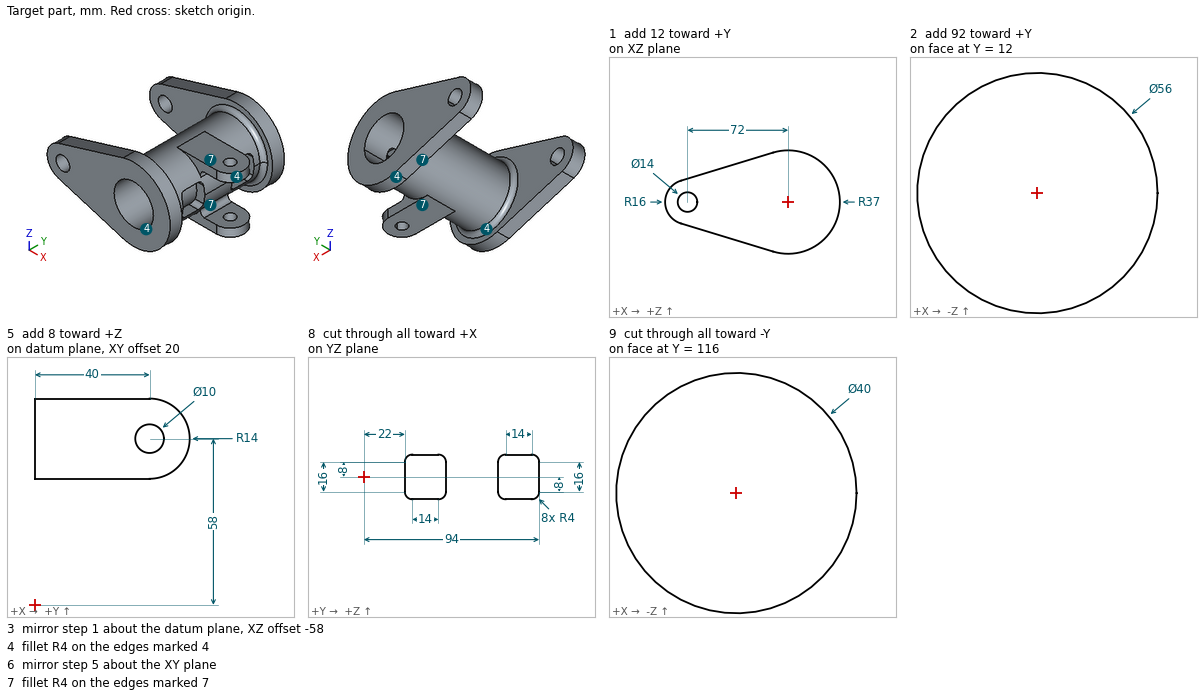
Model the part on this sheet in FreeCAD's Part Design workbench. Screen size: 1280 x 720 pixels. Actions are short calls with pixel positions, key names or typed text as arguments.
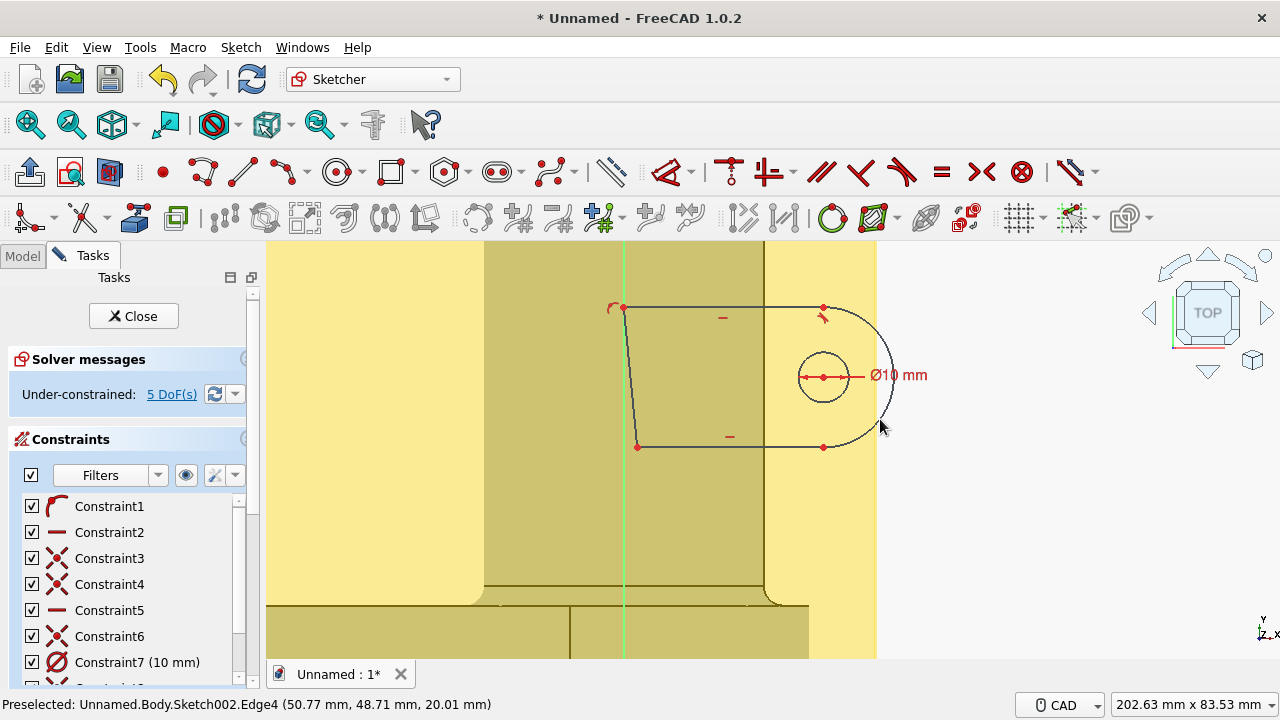
click(693, 447)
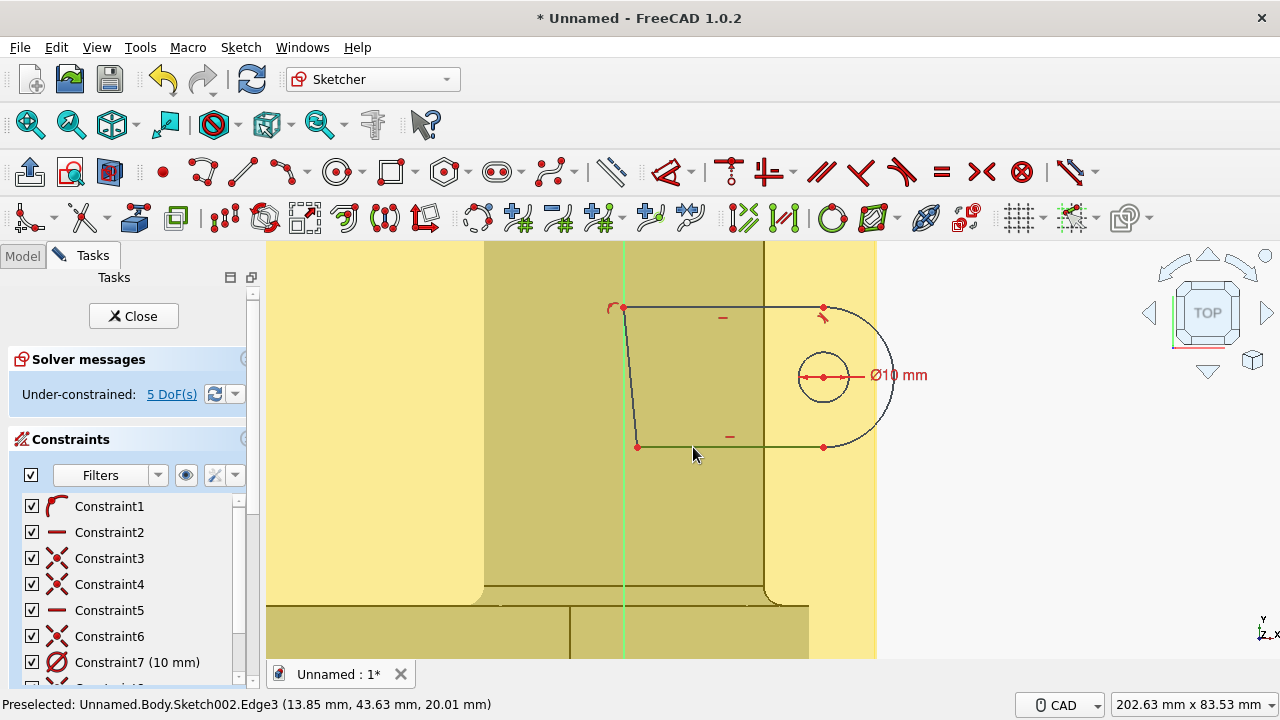
click(880, 419)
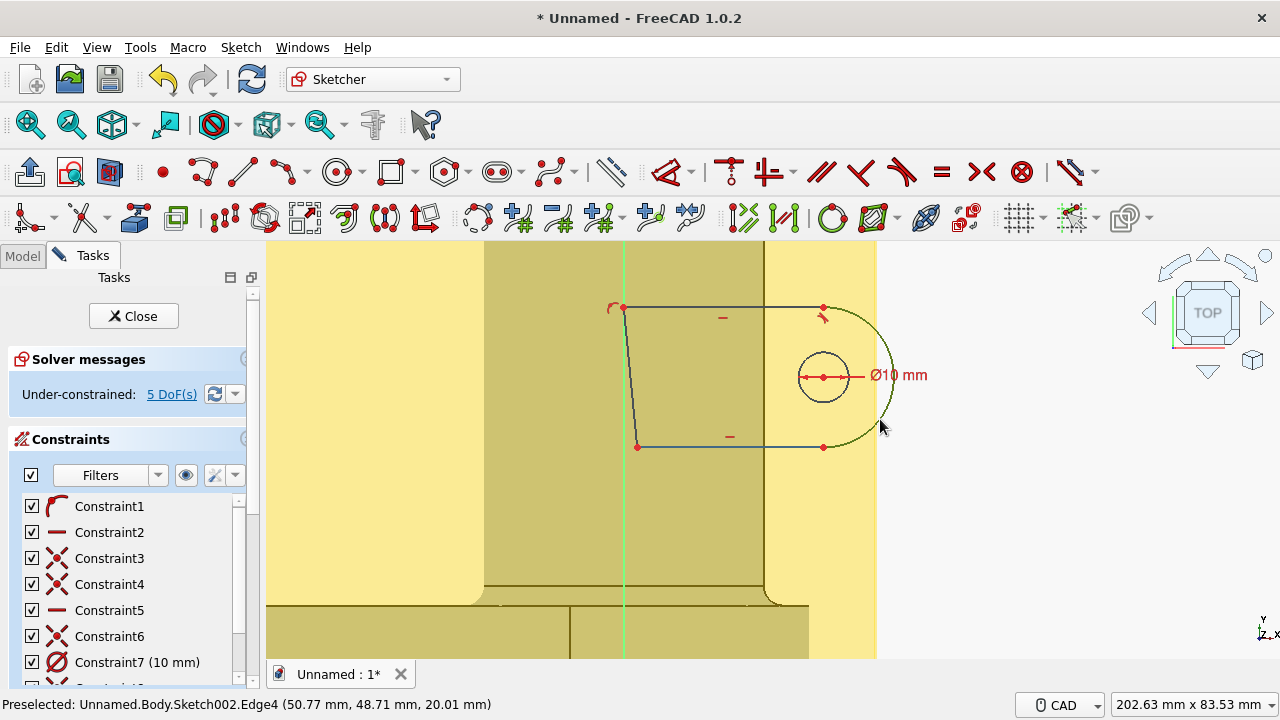
click(902, 172)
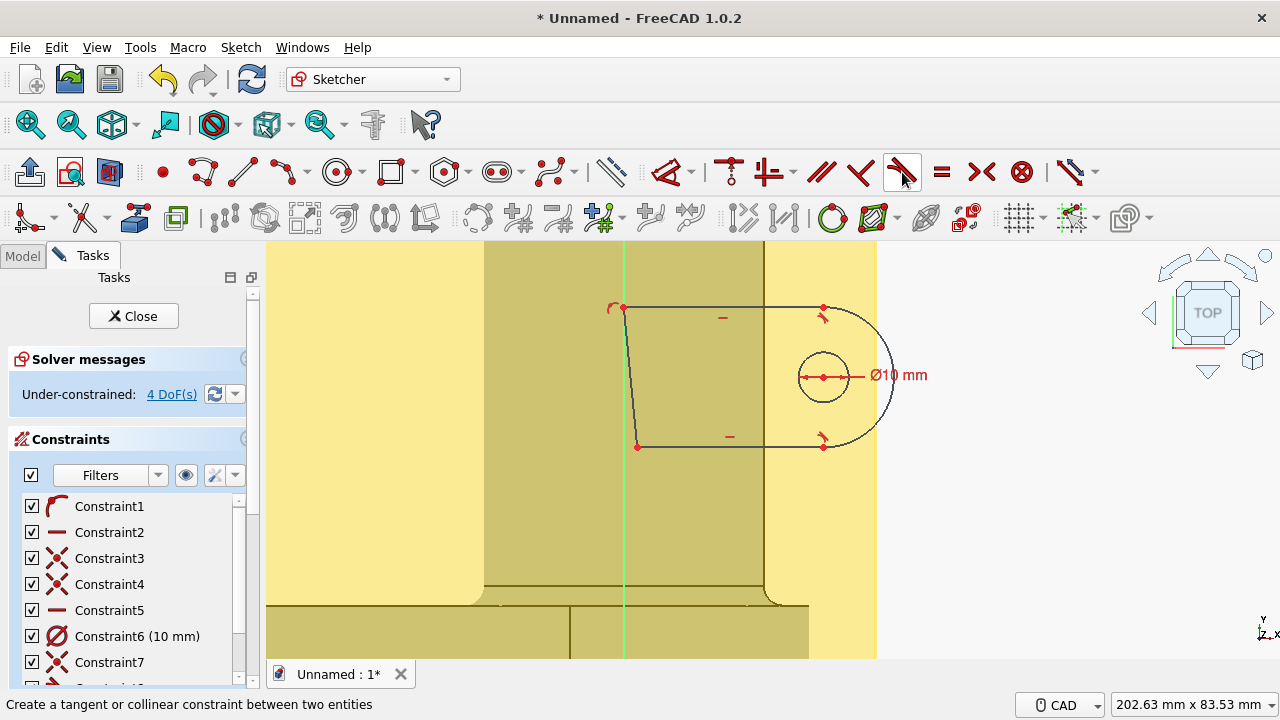
scroll(633, 405, up, 2)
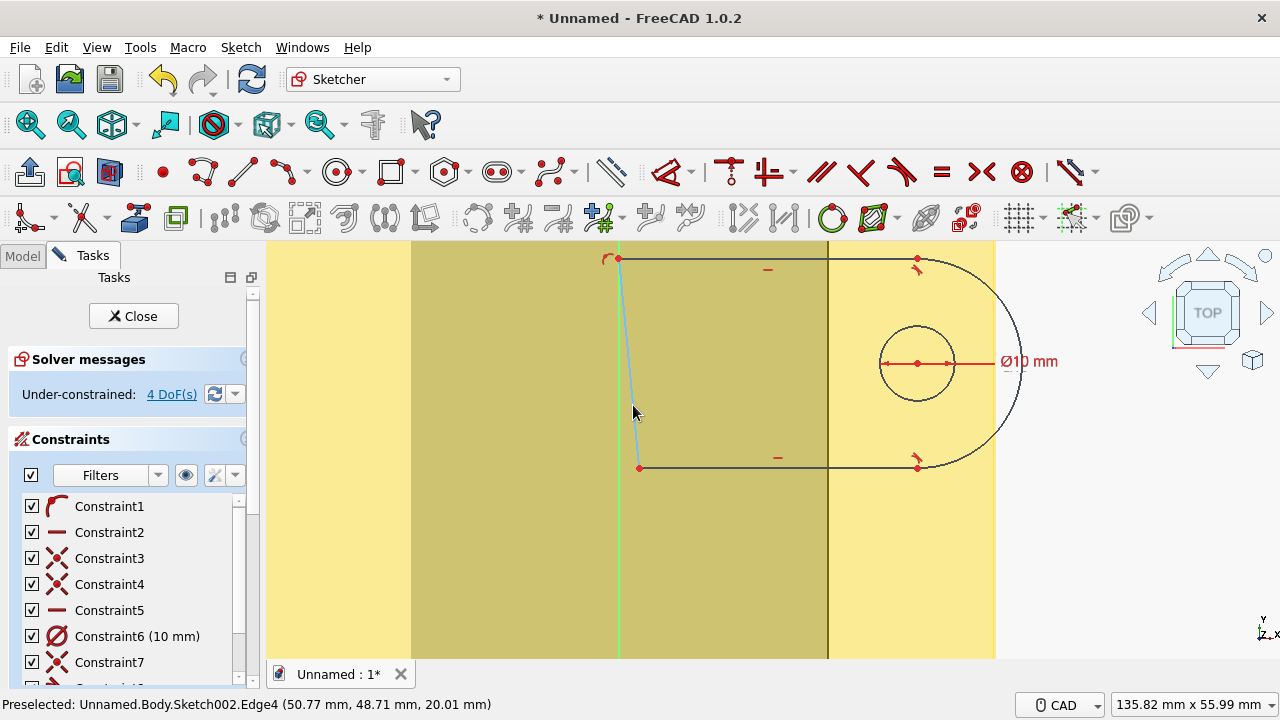
click(633, 405)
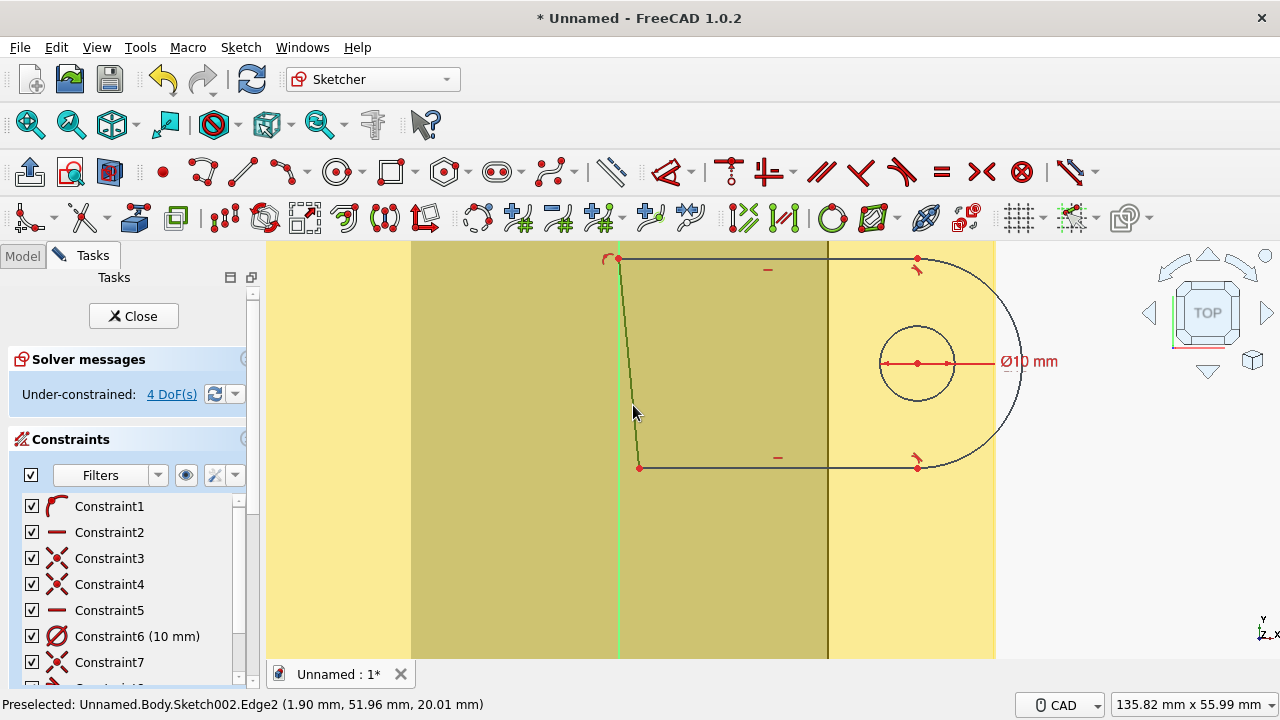
key(v)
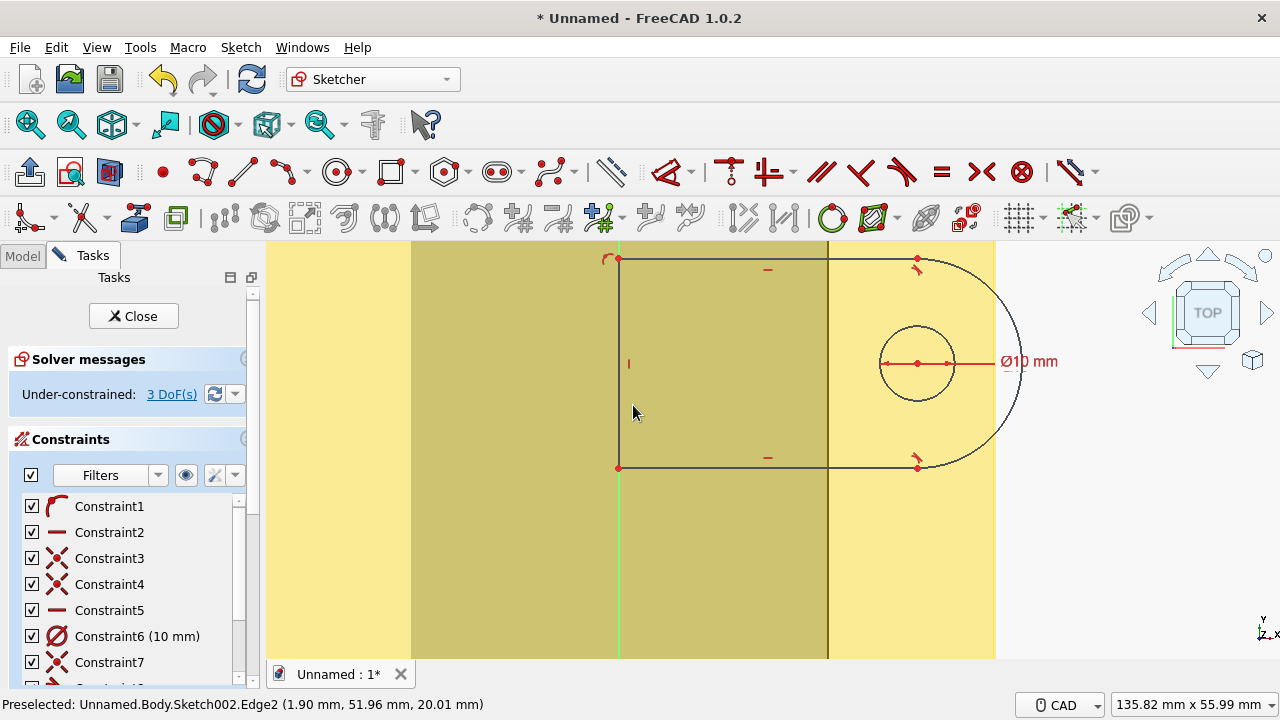
click(666, 172)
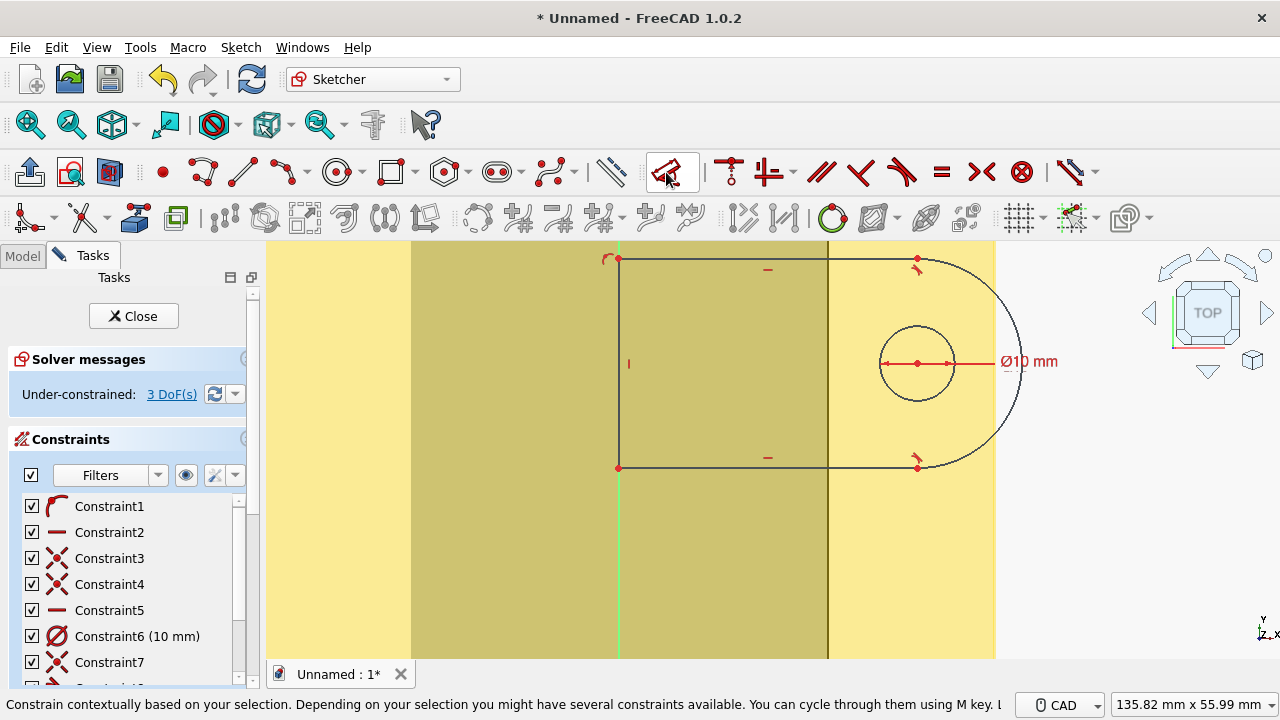
click(1002, 425)
click(1028, 444)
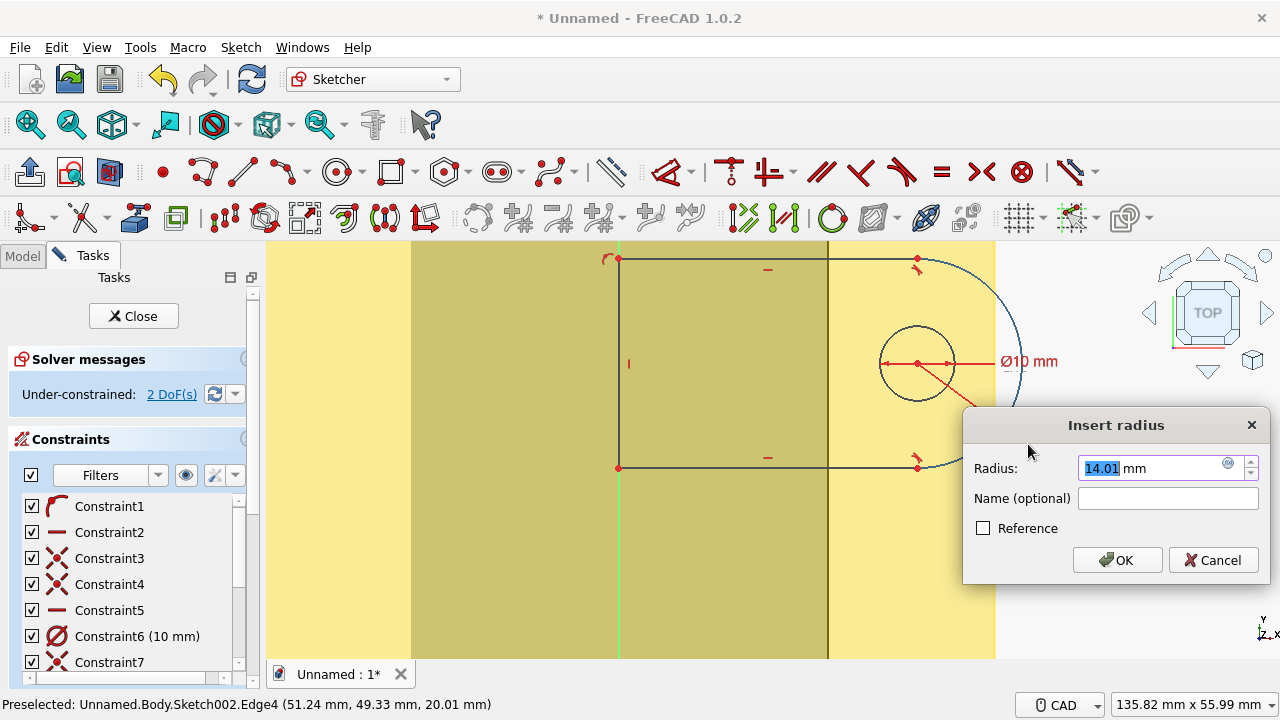
text(14)
key(Return)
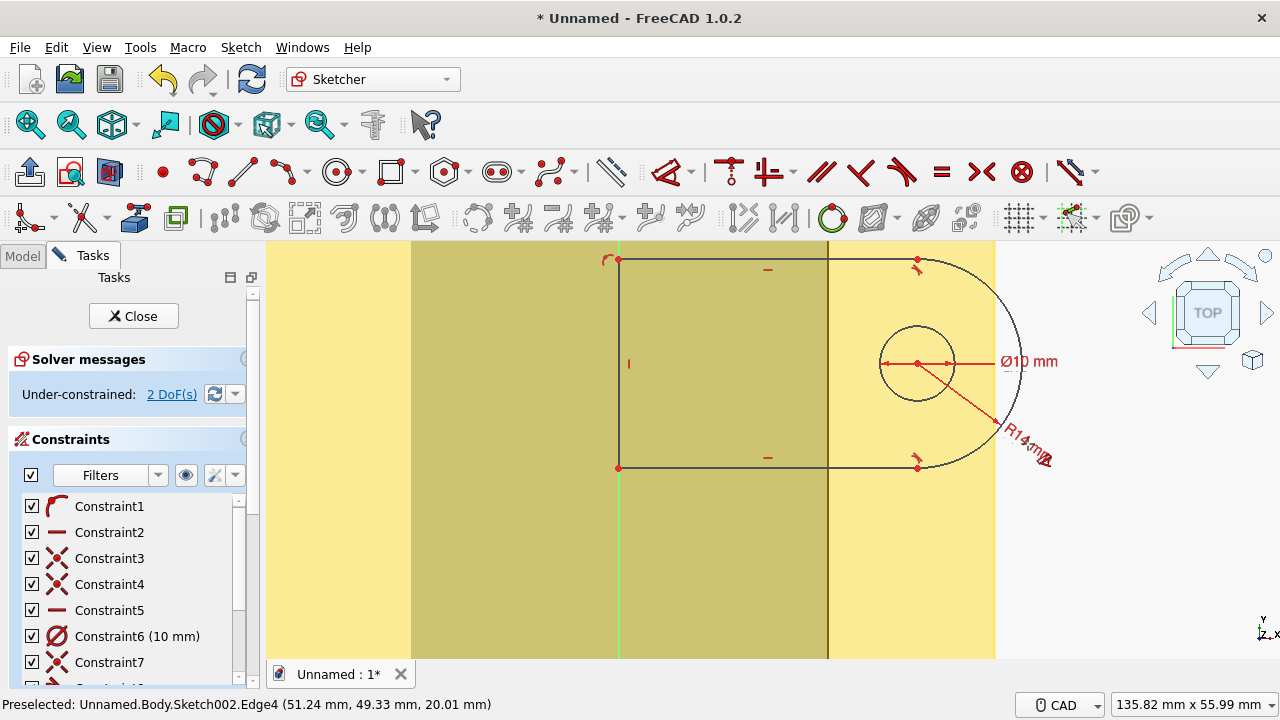
scroll(610, 389, down, 4)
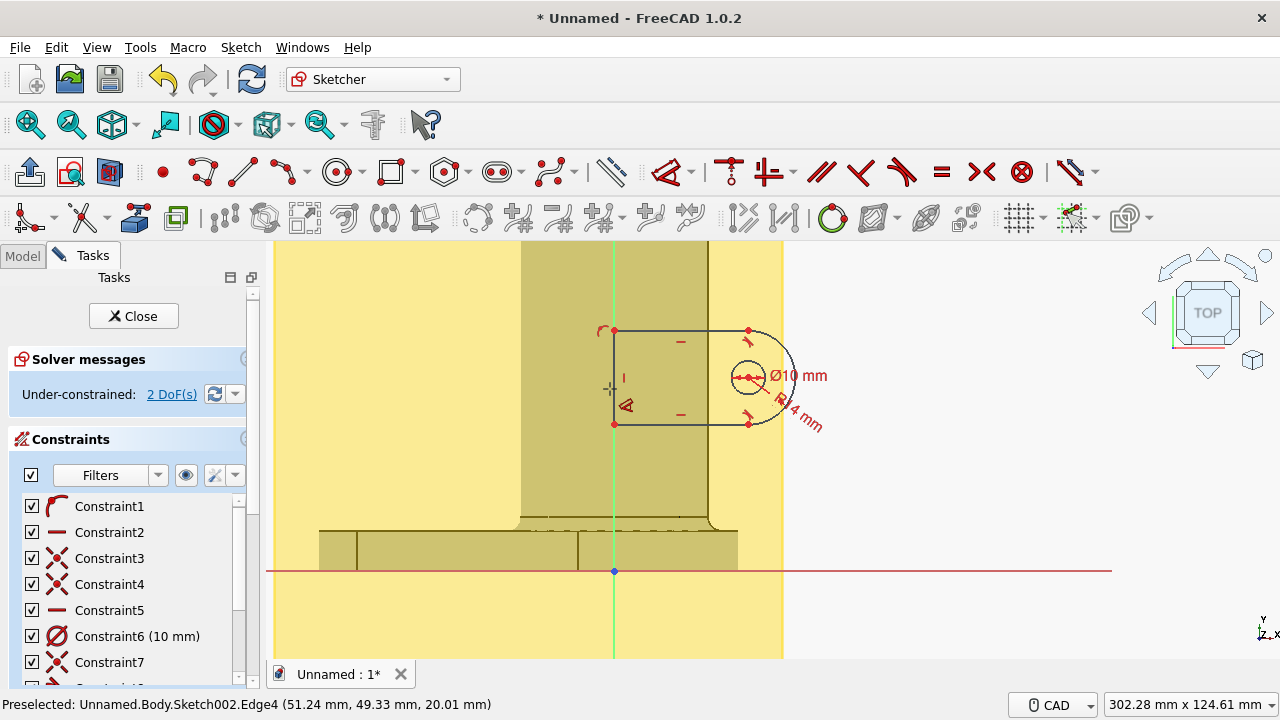
click(708, 331)
click(681, 297)